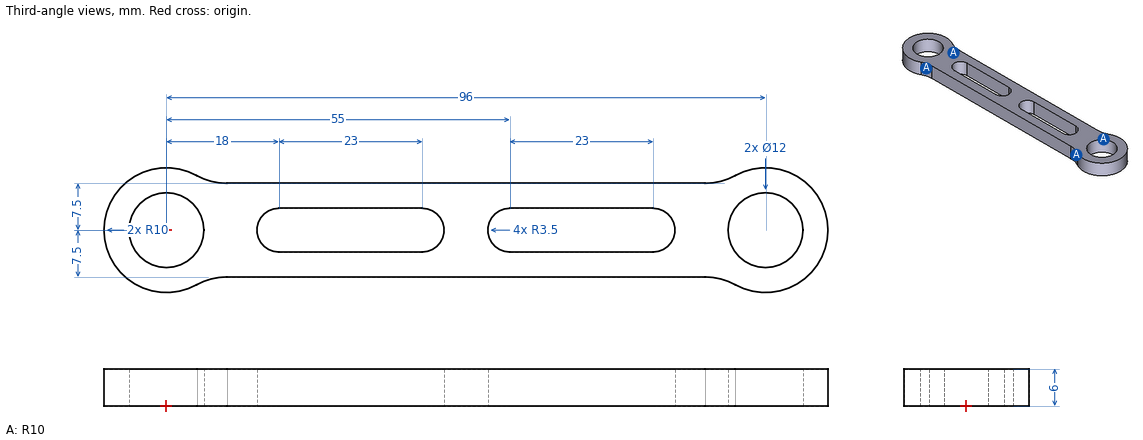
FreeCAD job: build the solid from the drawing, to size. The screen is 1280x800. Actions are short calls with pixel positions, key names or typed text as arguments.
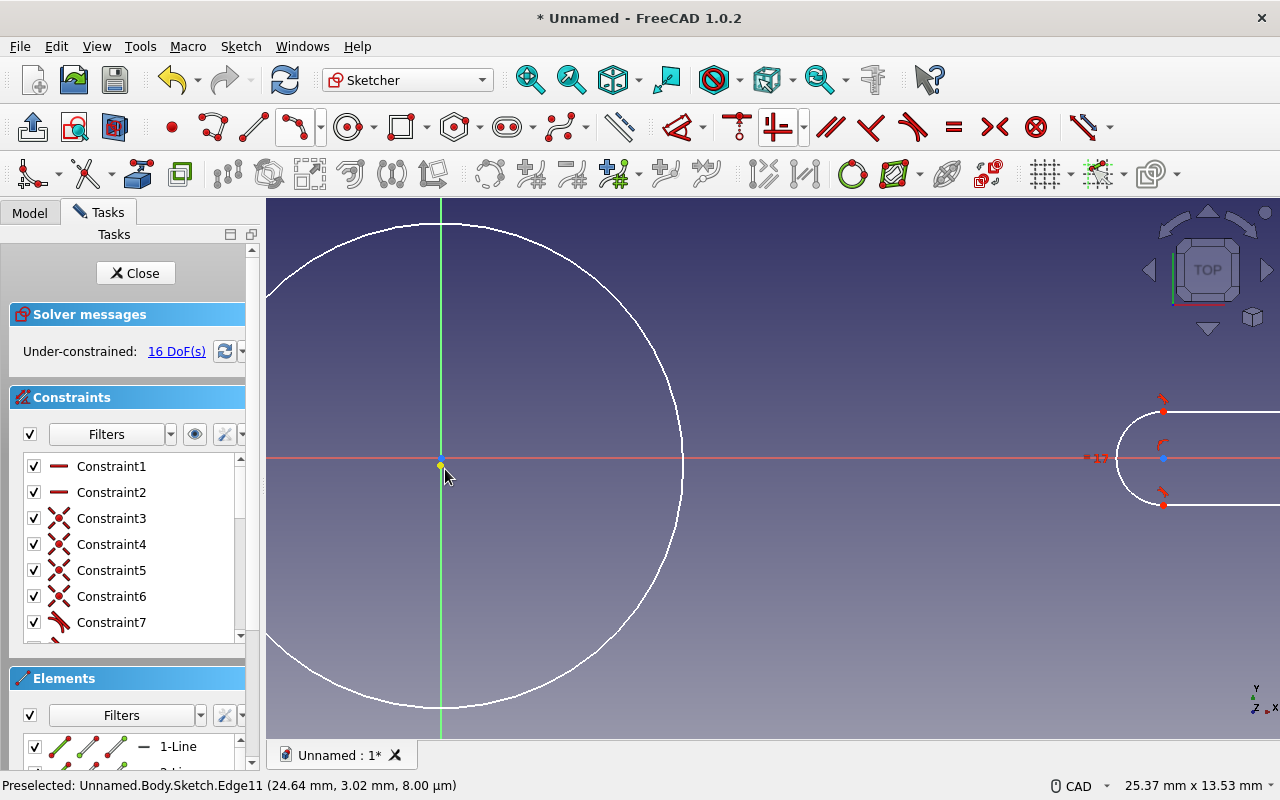
drag(431, 448, 451, 476)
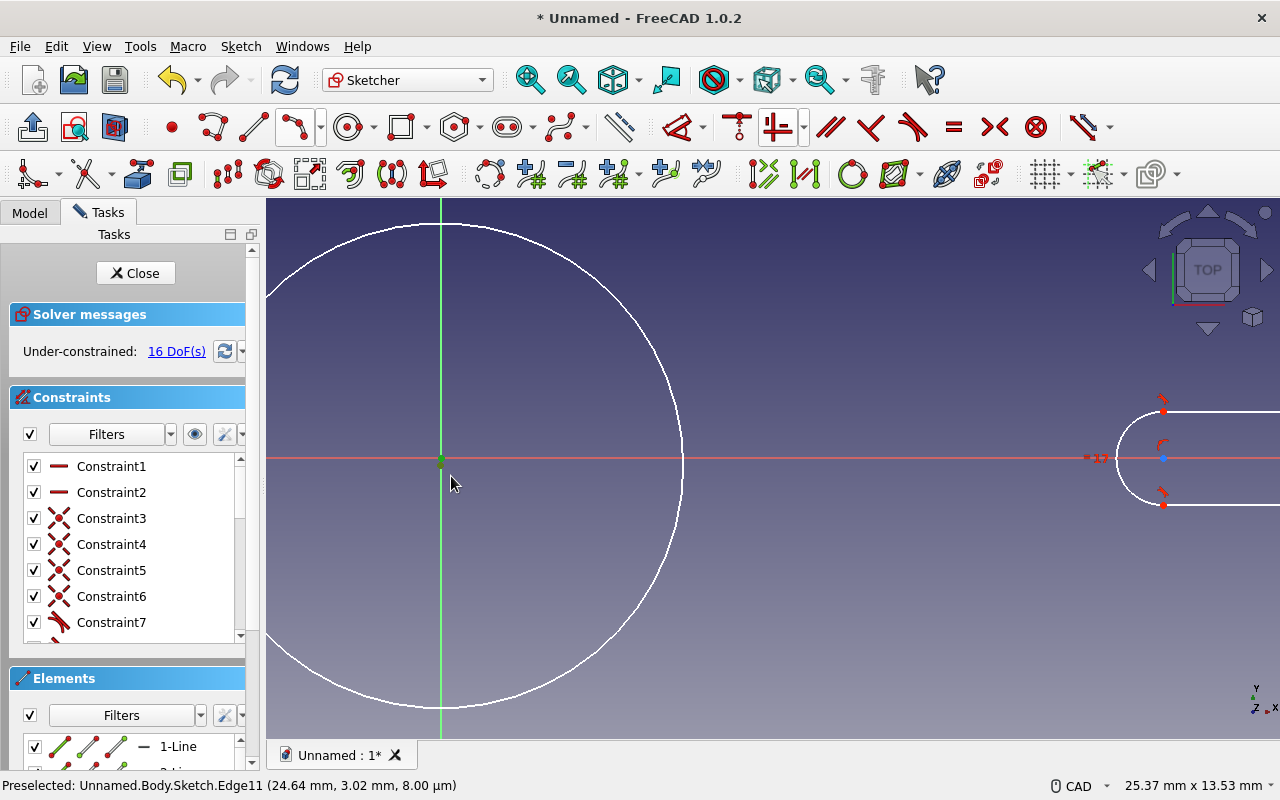
click(737, 128)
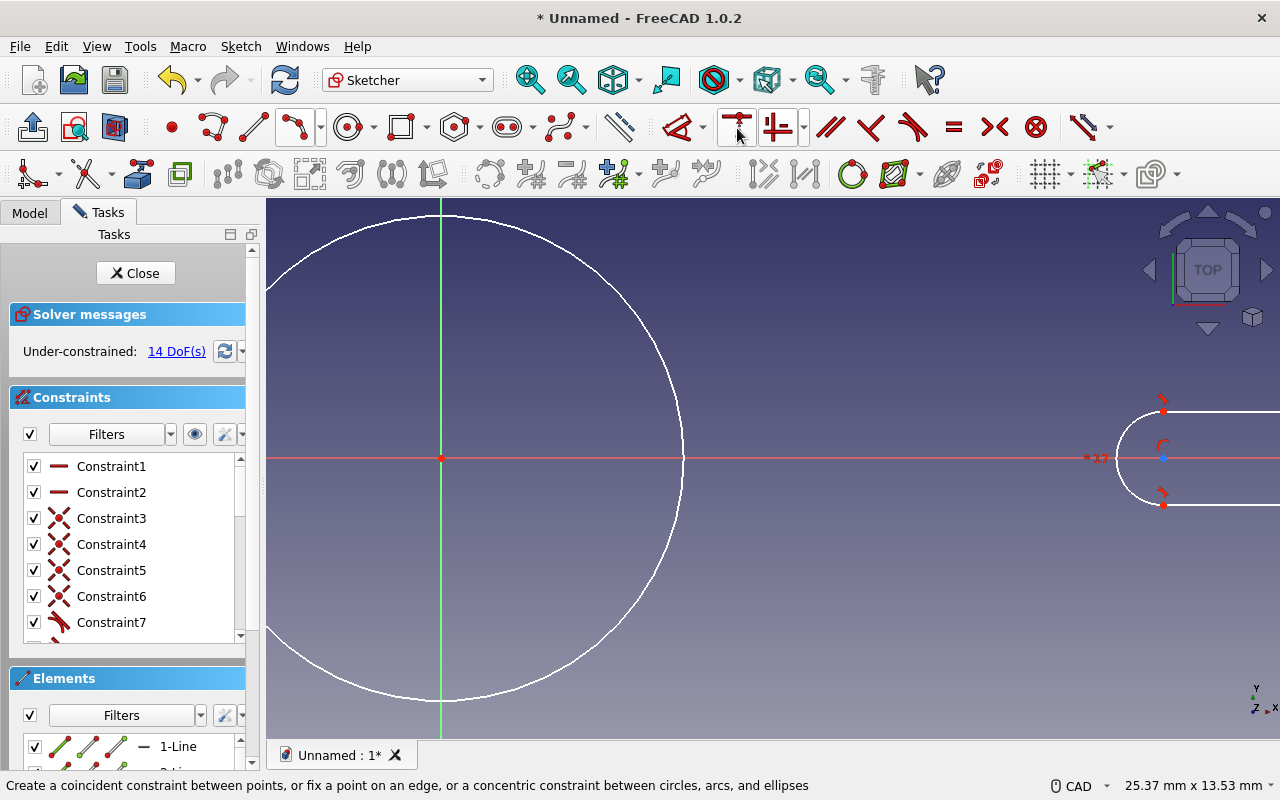
scroll(445, 470, down, 10)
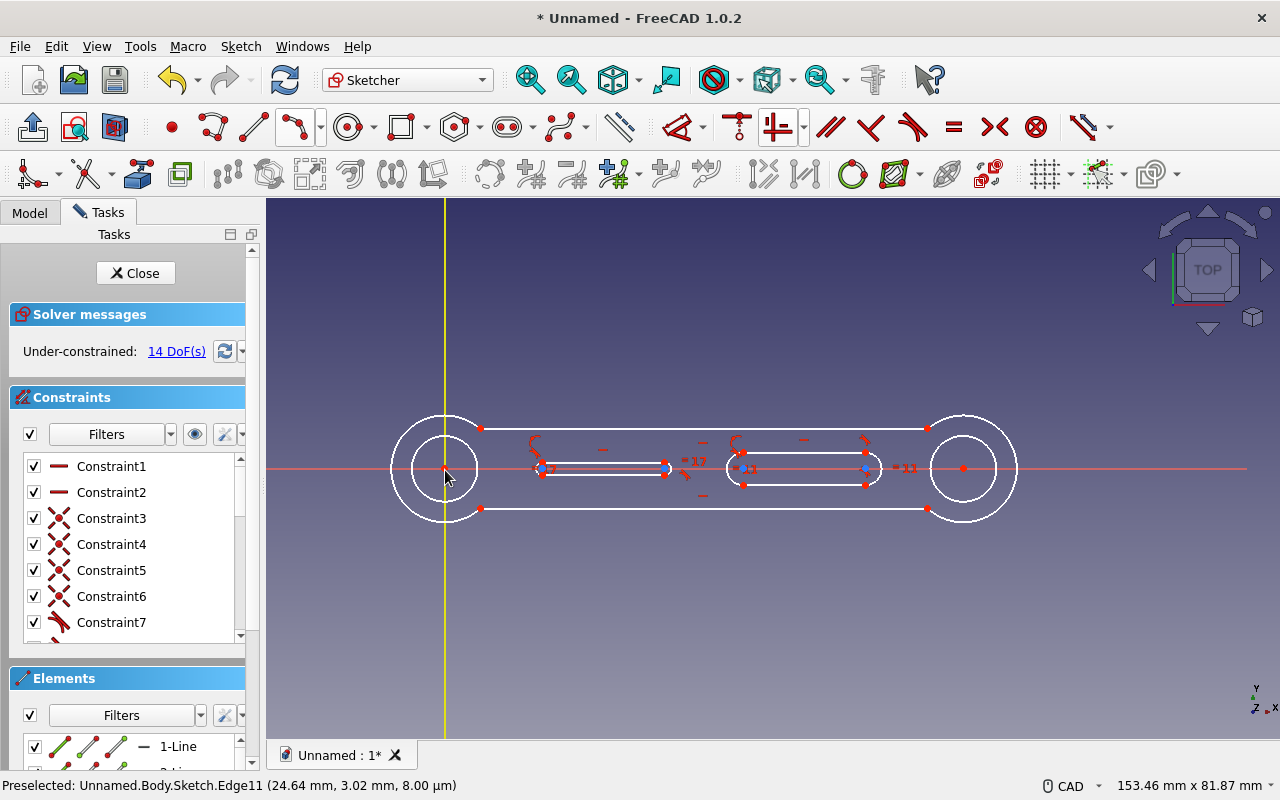
click(412, 426)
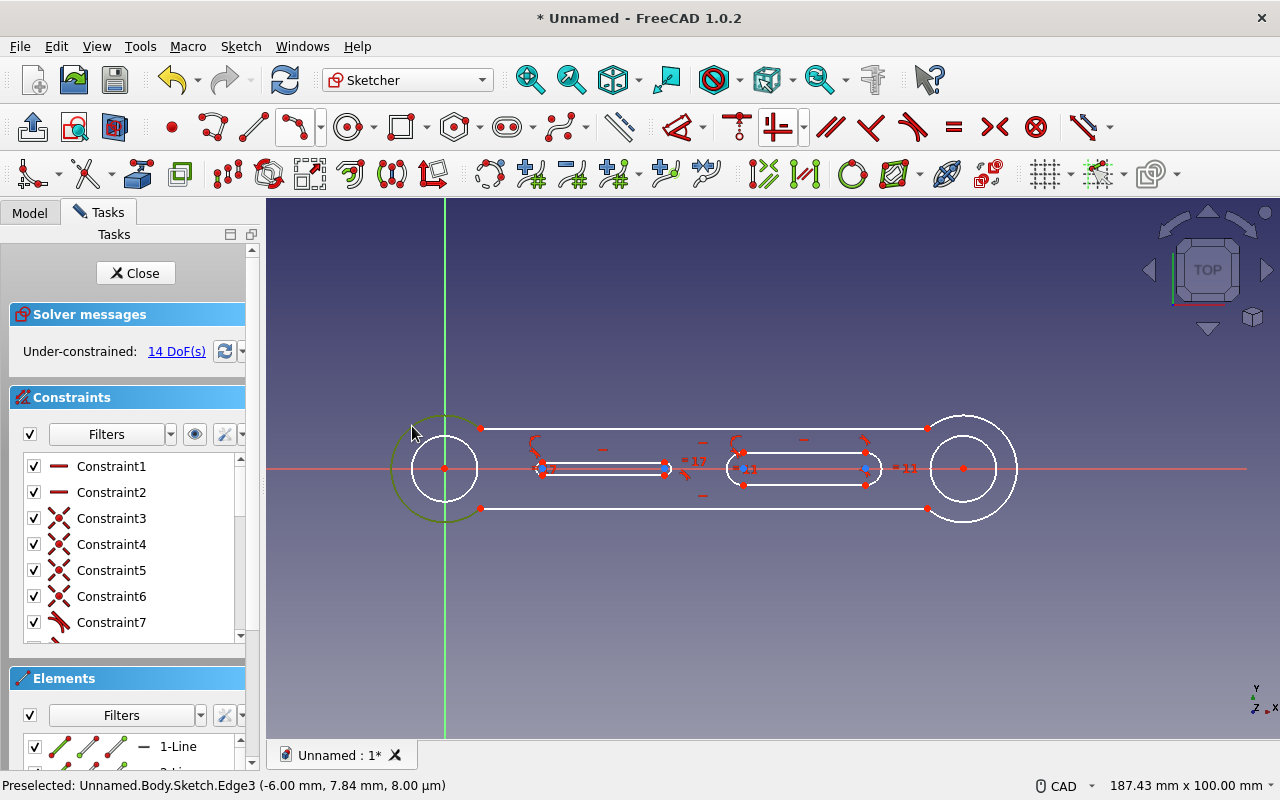
click(996, 511)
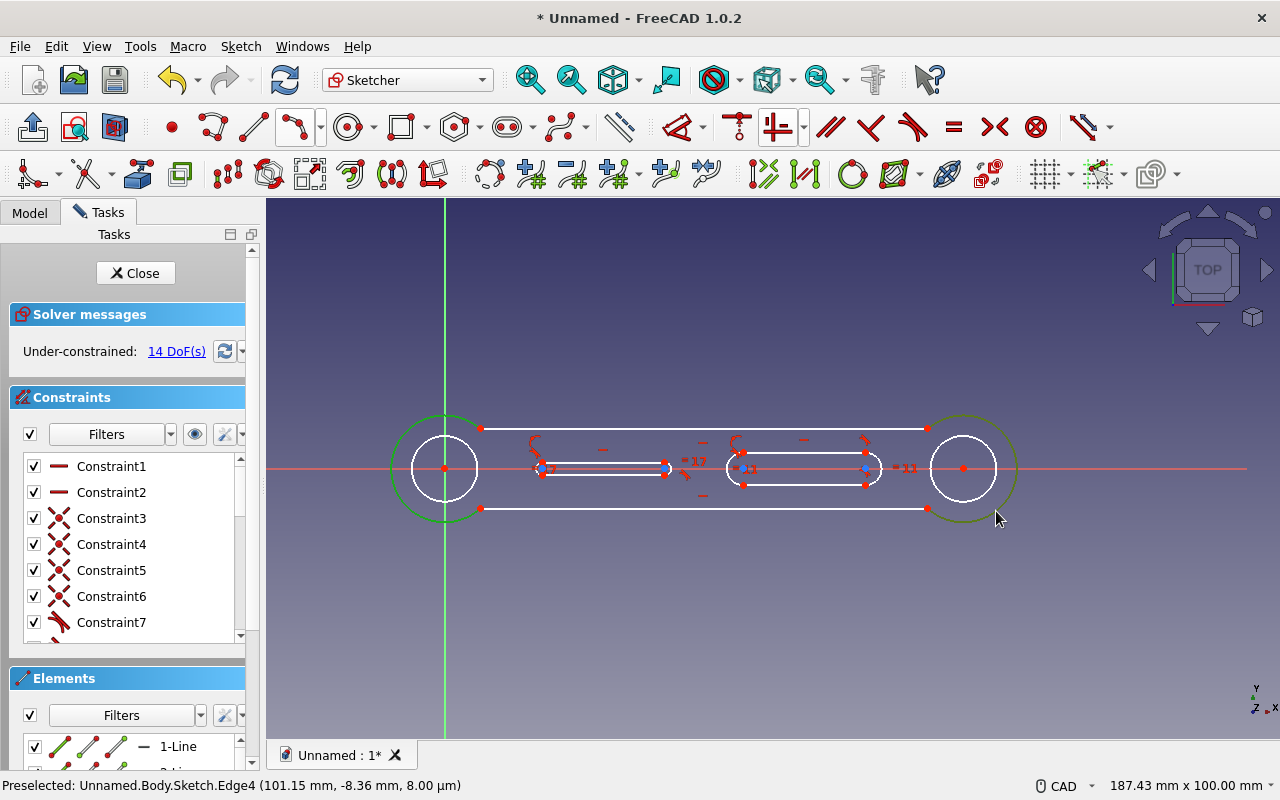
key(e)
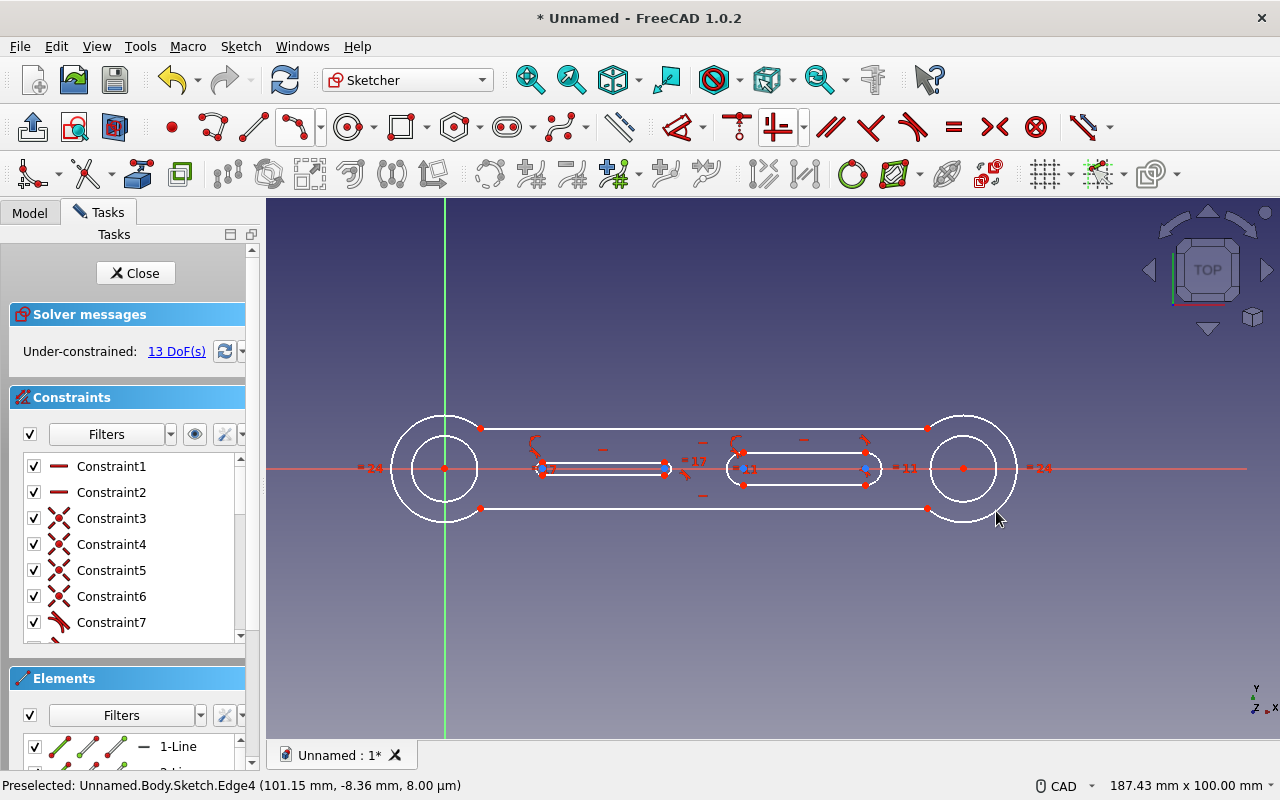
scroll(730, 459, up, 2)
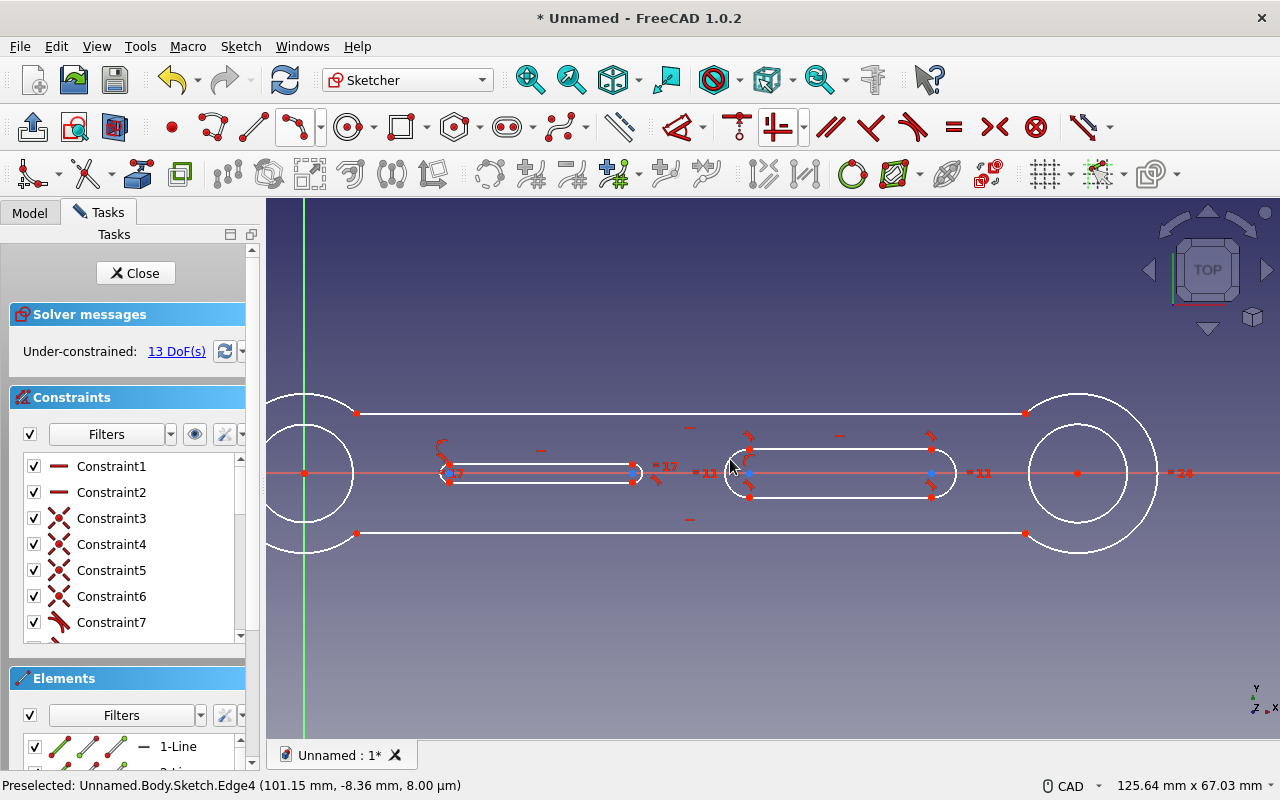
click(730, 459)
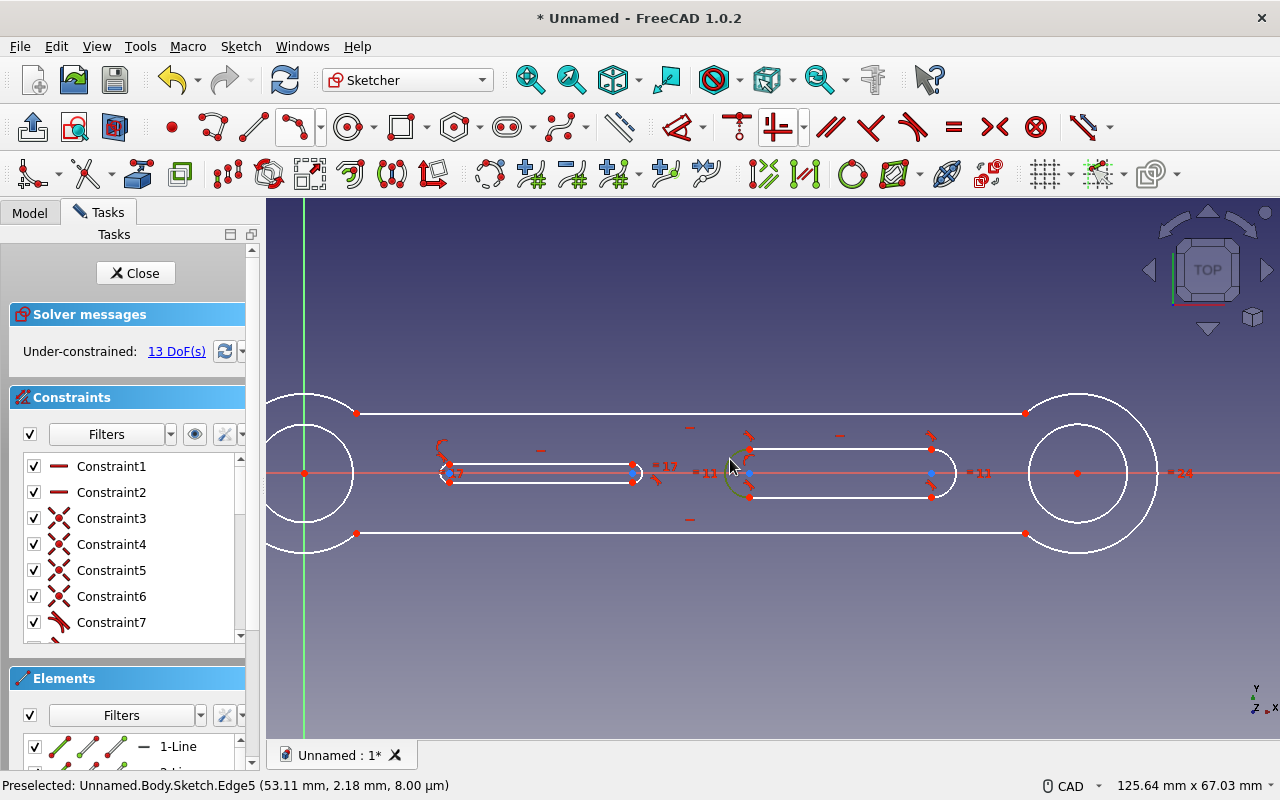
scroll(440, 473, up, 2)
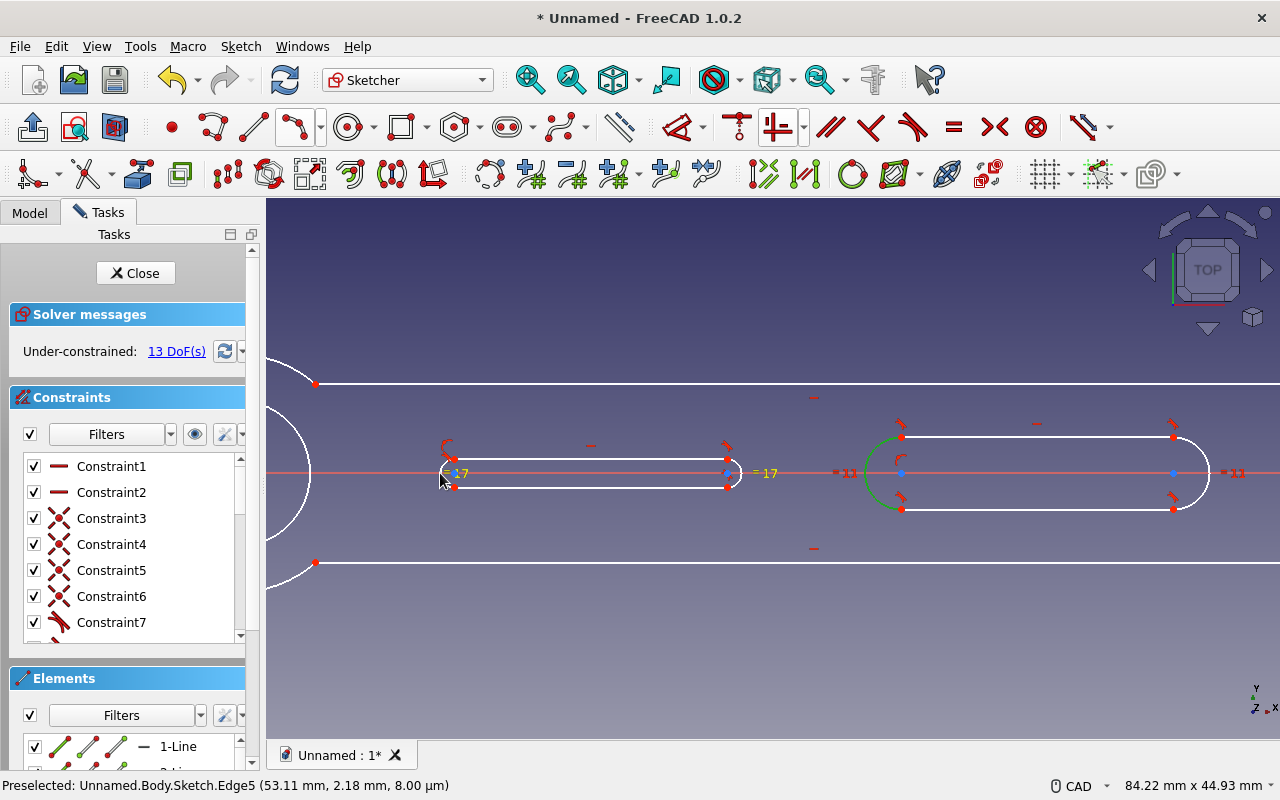
click(441, 473)